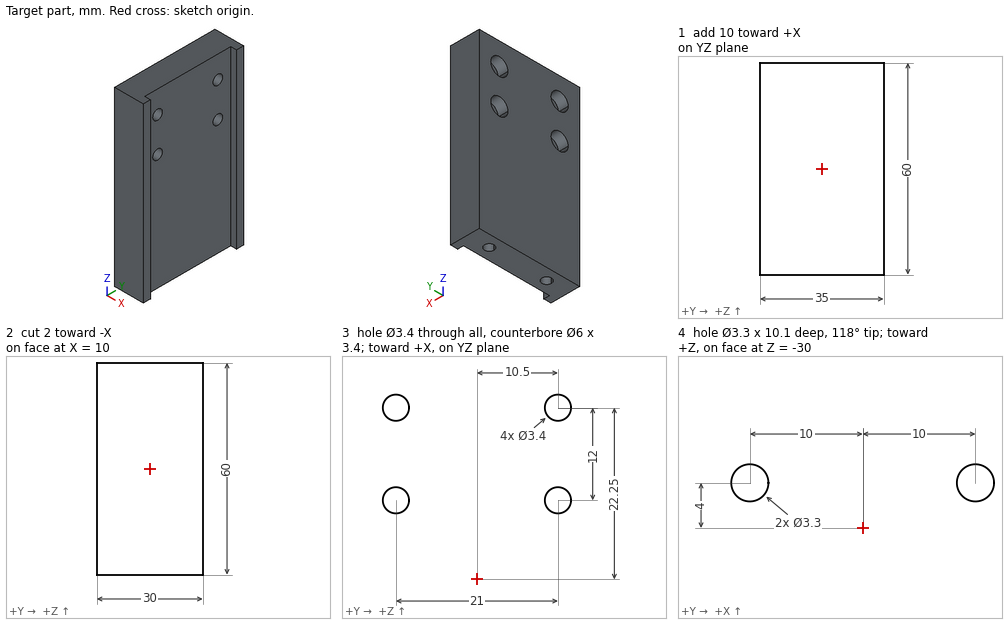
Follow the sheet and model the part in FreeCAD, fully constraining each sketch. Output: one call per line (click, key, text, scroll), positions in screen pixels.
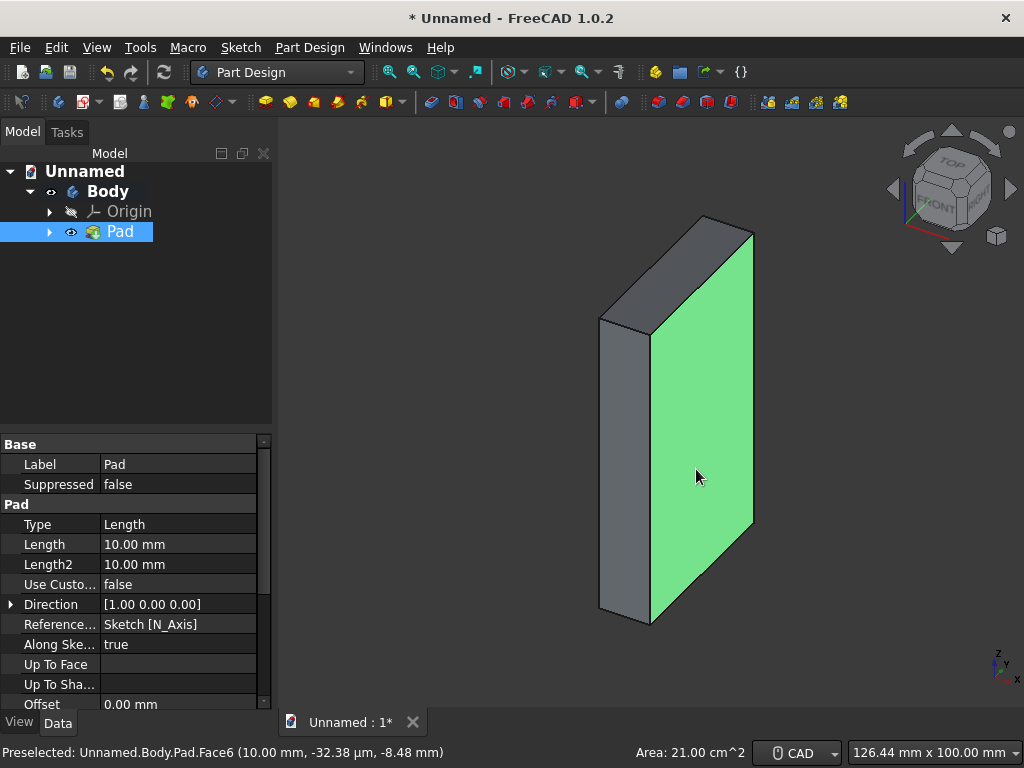
click(84, 102)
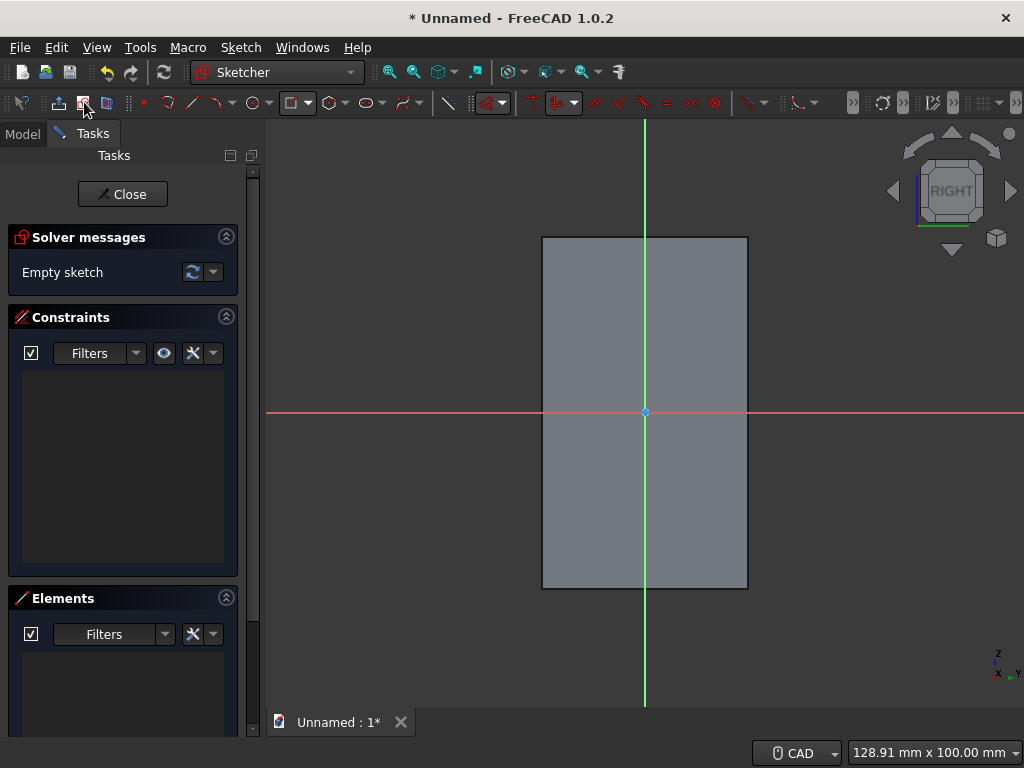
click(292, 104)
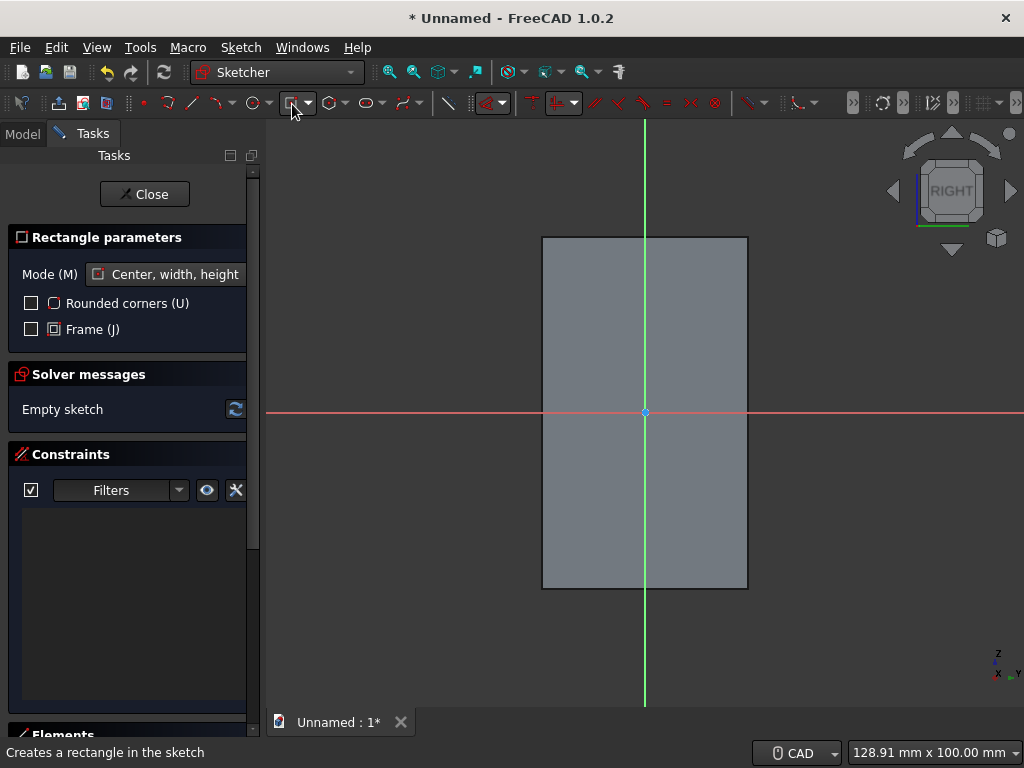
click(645, 413)
move(733, 237)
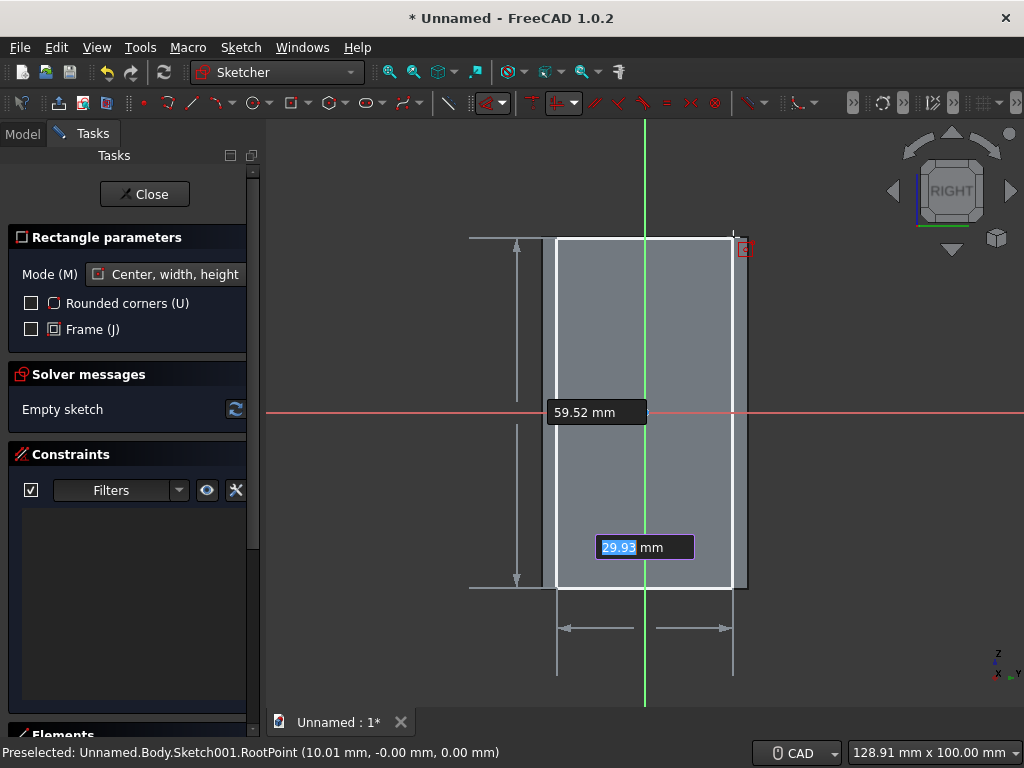
text(30)
key(Tab)
text(60)
key(Return)
key(Escape)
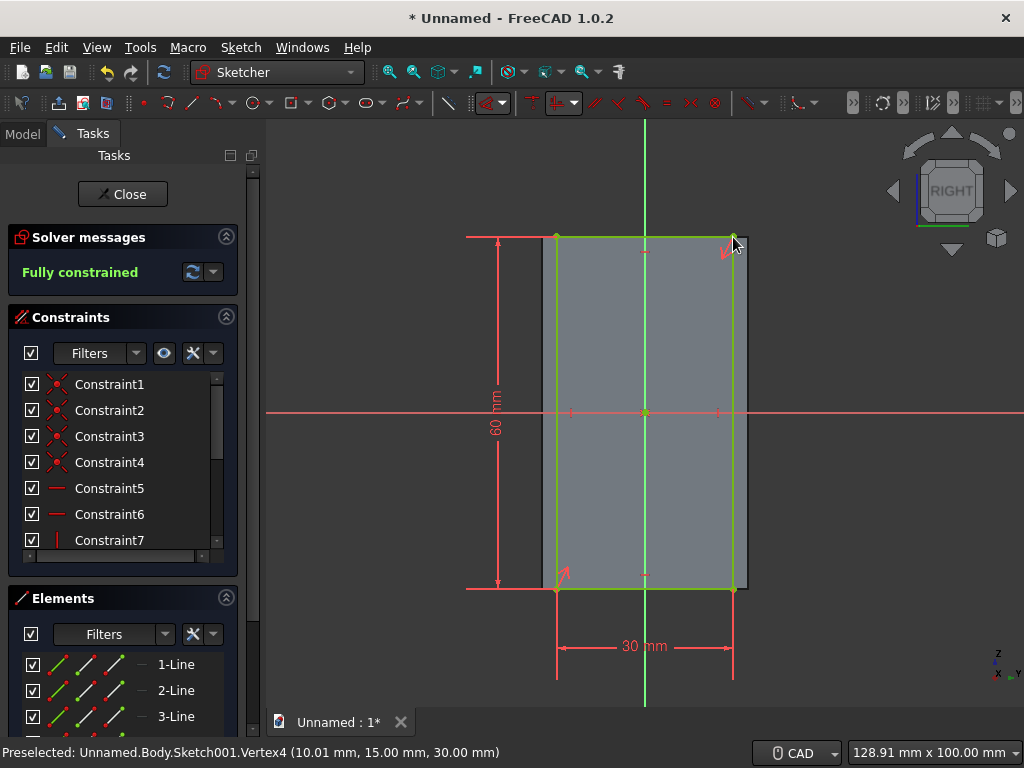
click(123, 194)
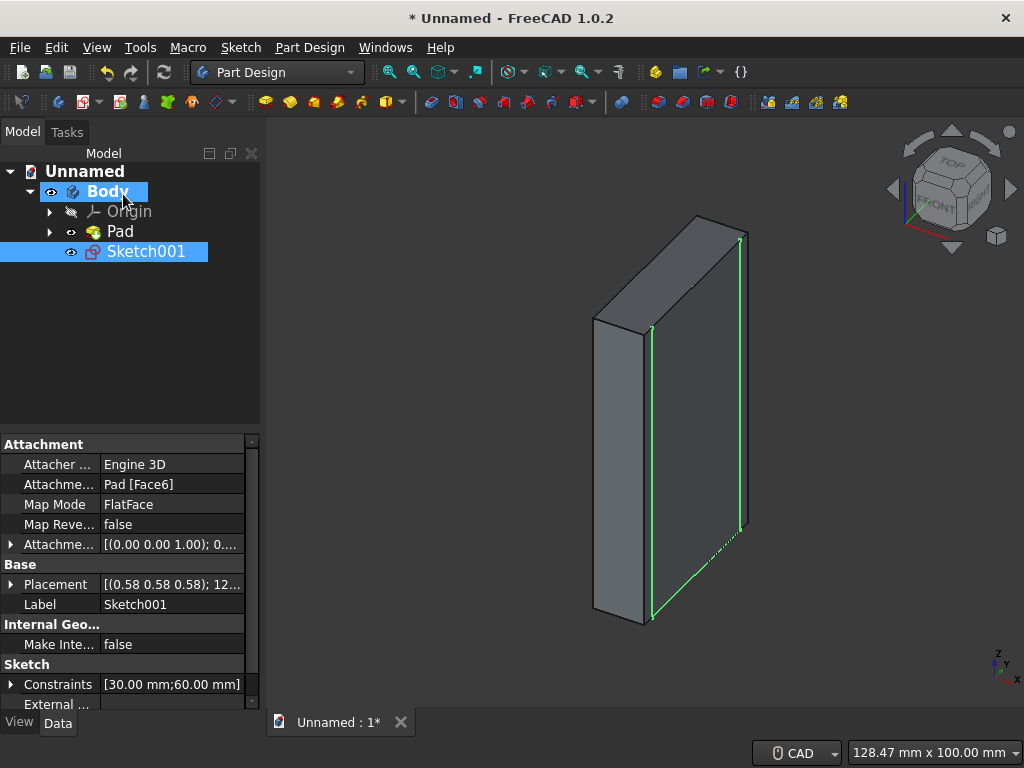
click(432, 102)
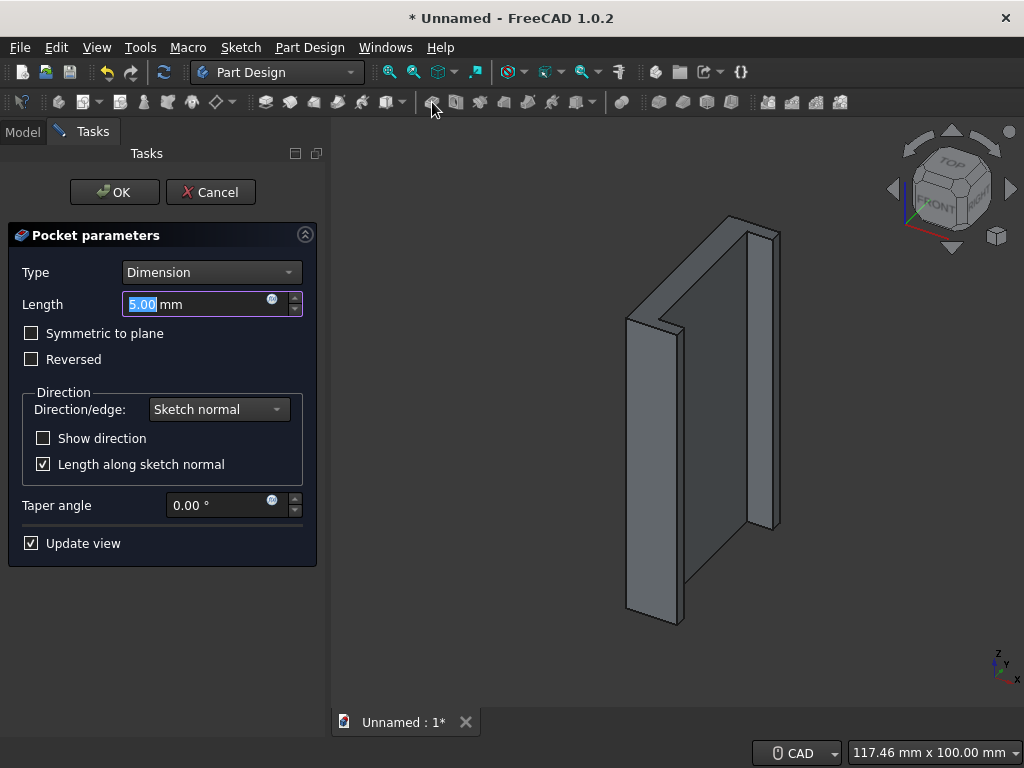
text(2)
key(Tab)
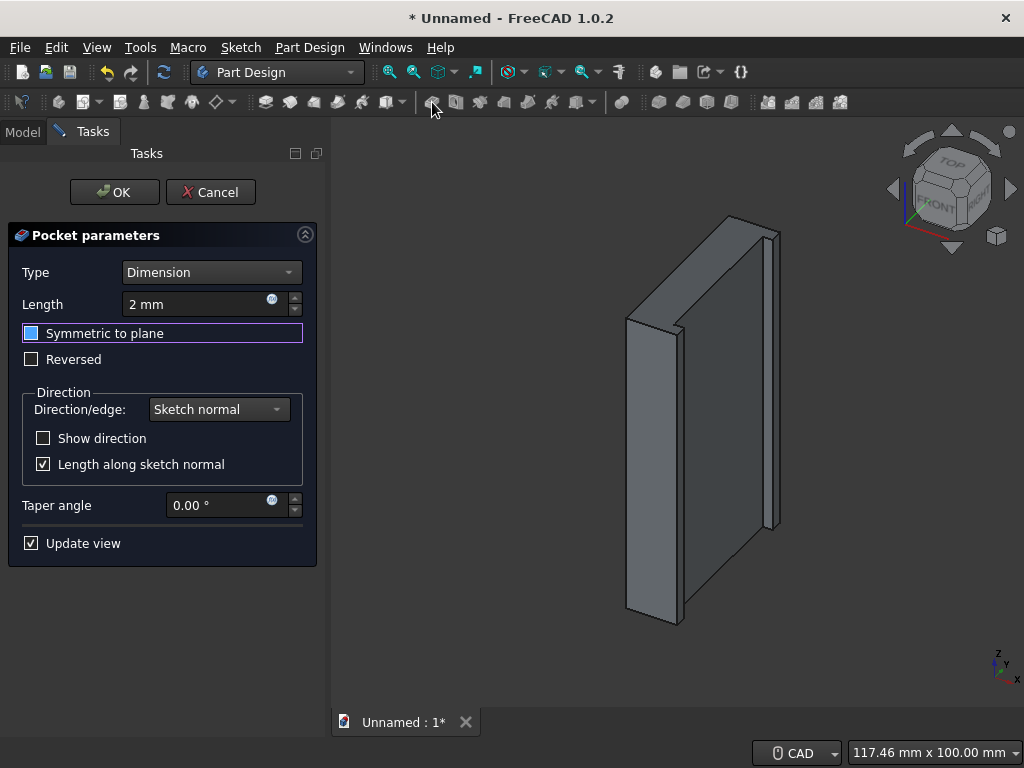
click(115, 192)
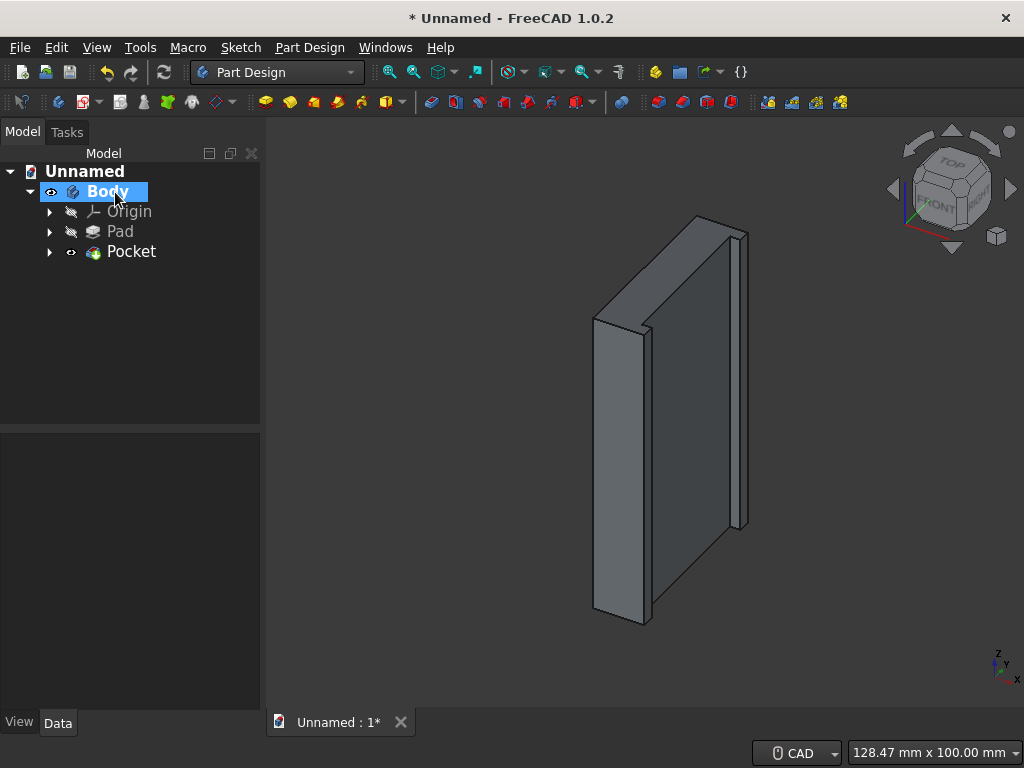
click(84, 102)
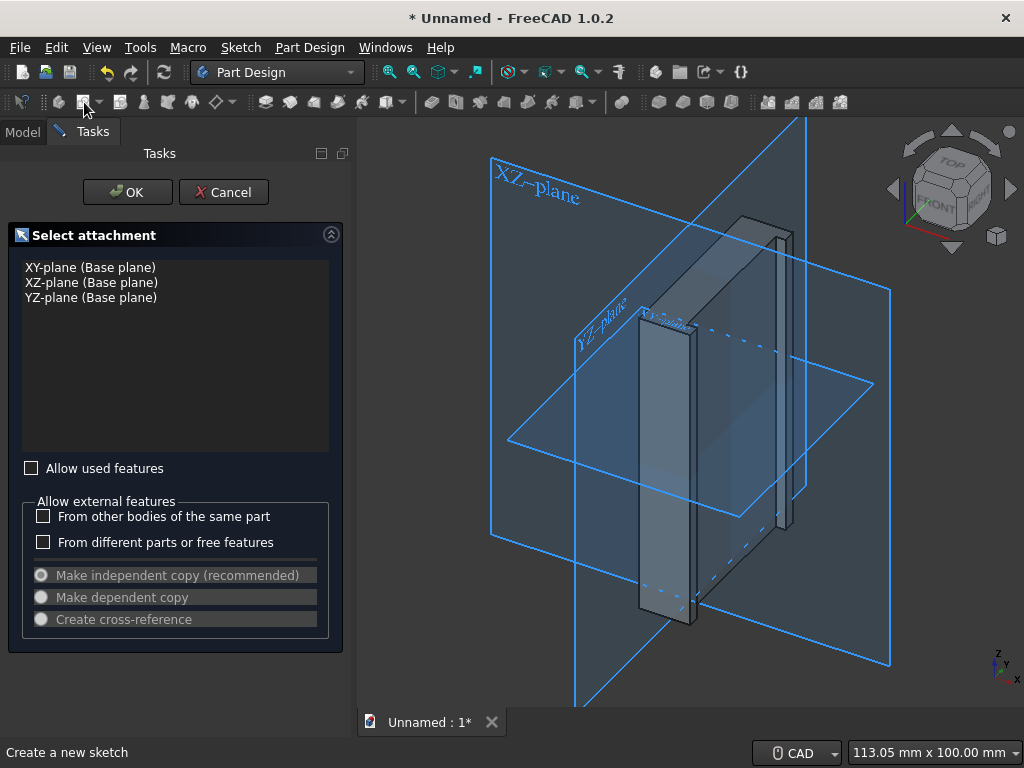
click(82, 298)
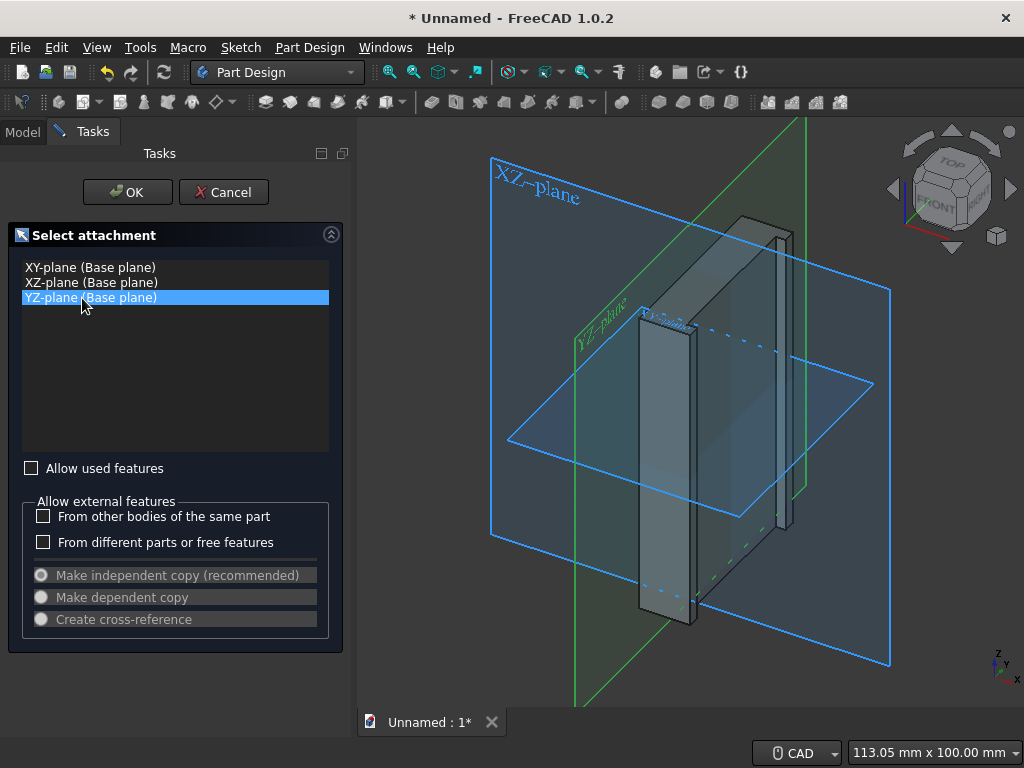
click(128, 192)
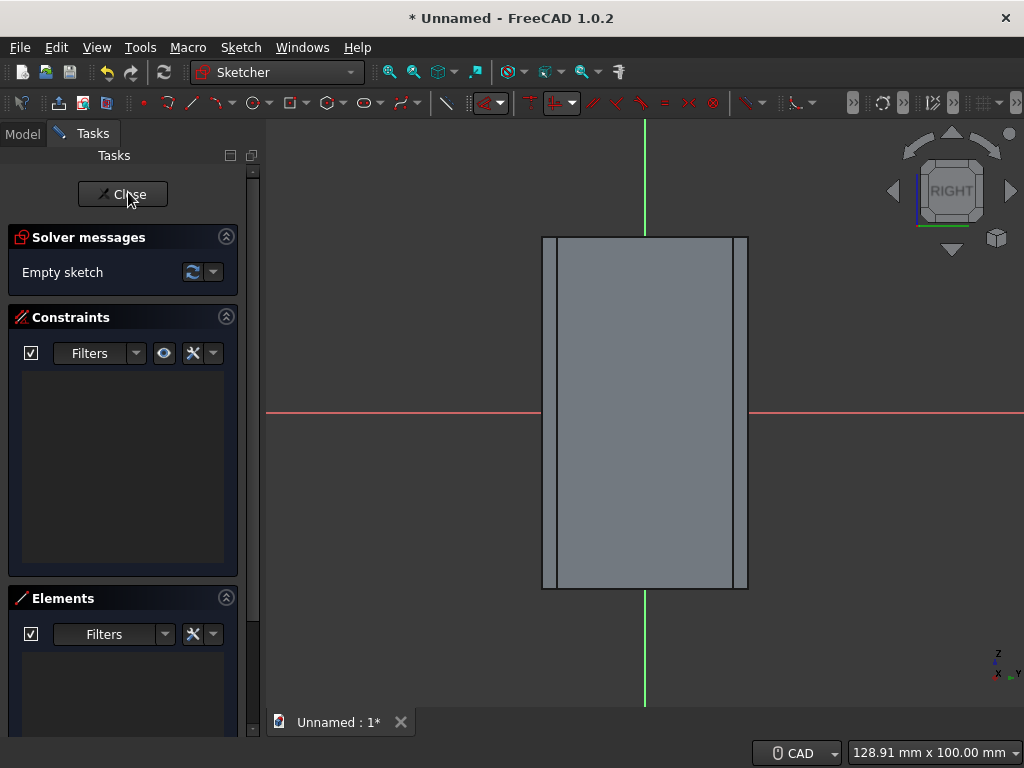
click(108, 104)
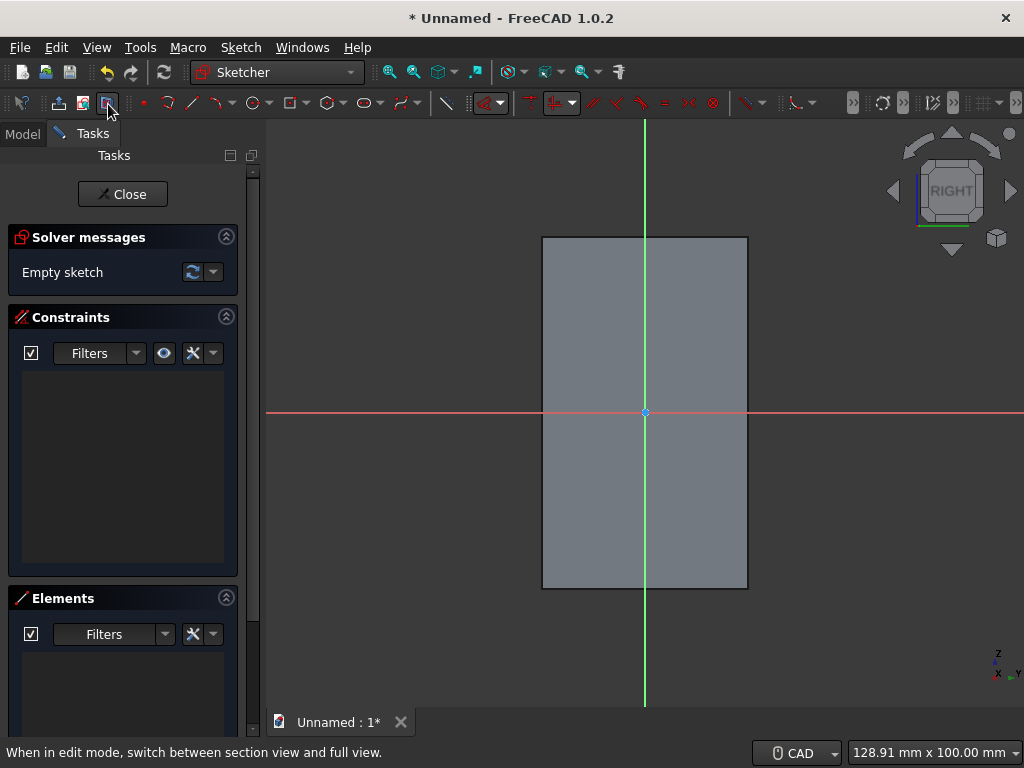
scroll(685, 302, up, 5)